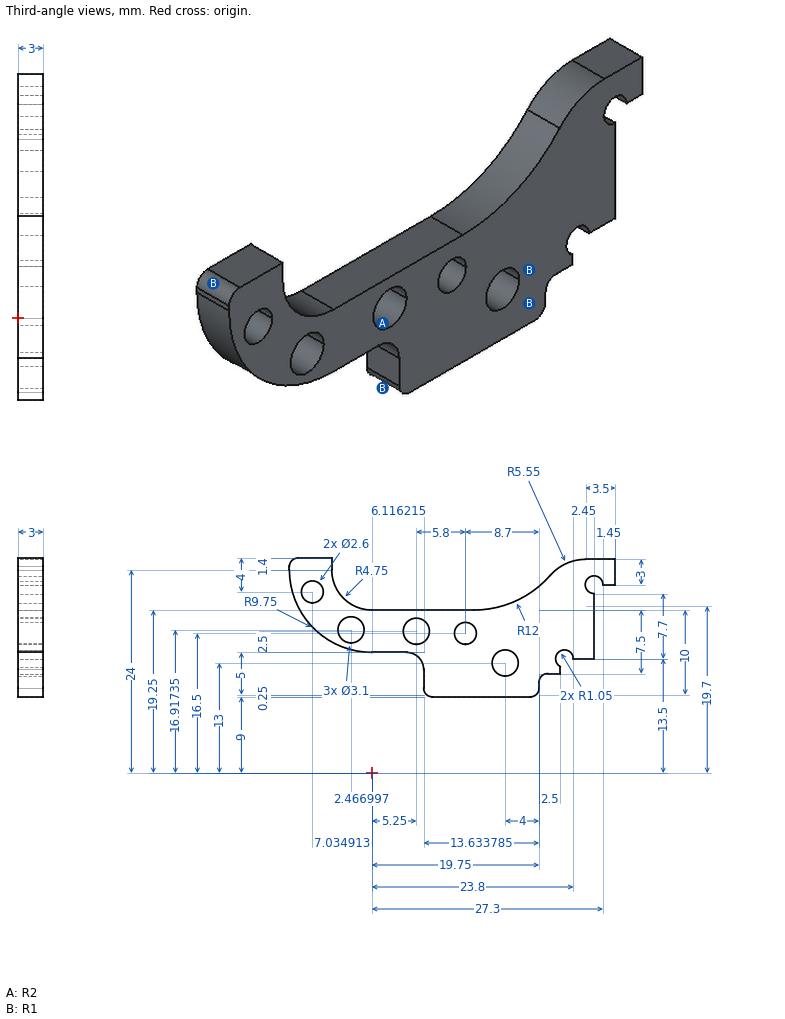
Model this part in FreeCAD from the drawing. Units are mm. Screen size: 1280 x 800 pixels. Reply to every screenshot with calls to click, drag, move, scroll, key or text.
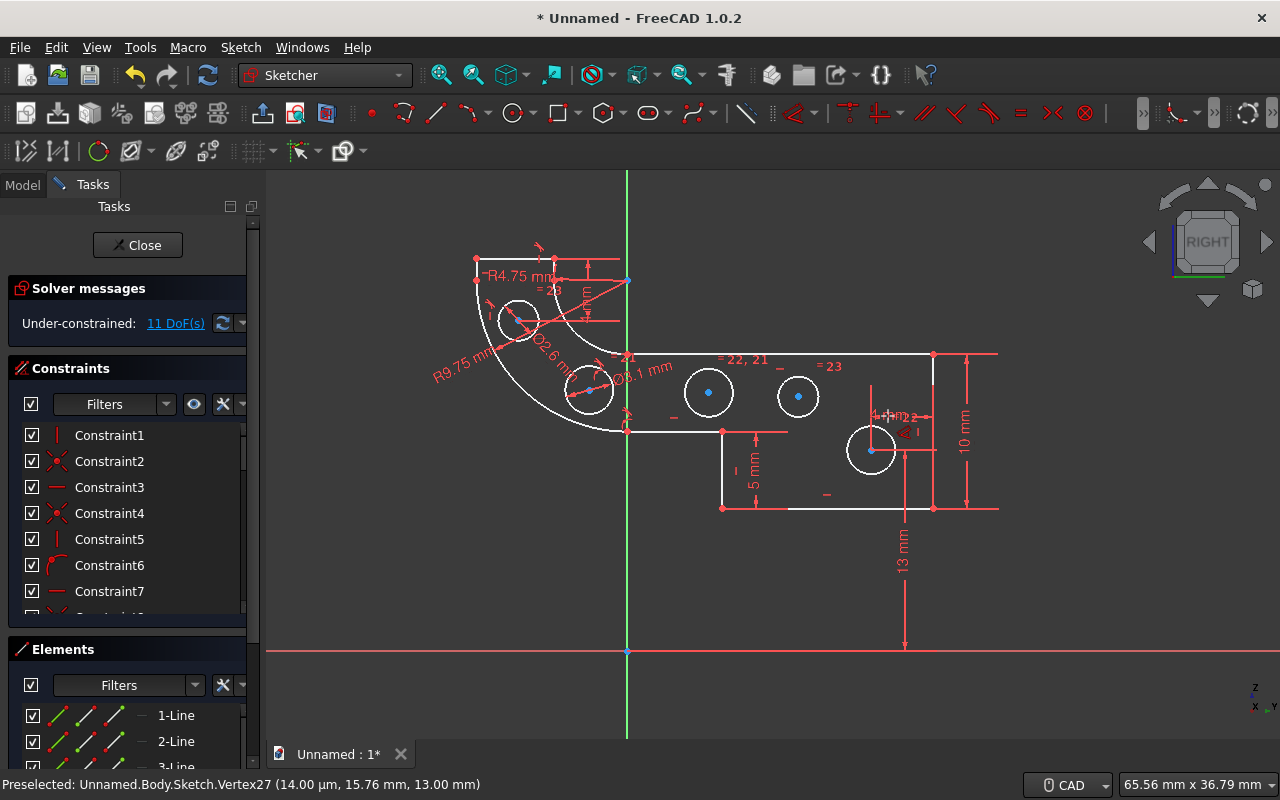
scroll(554, 270, up, 4)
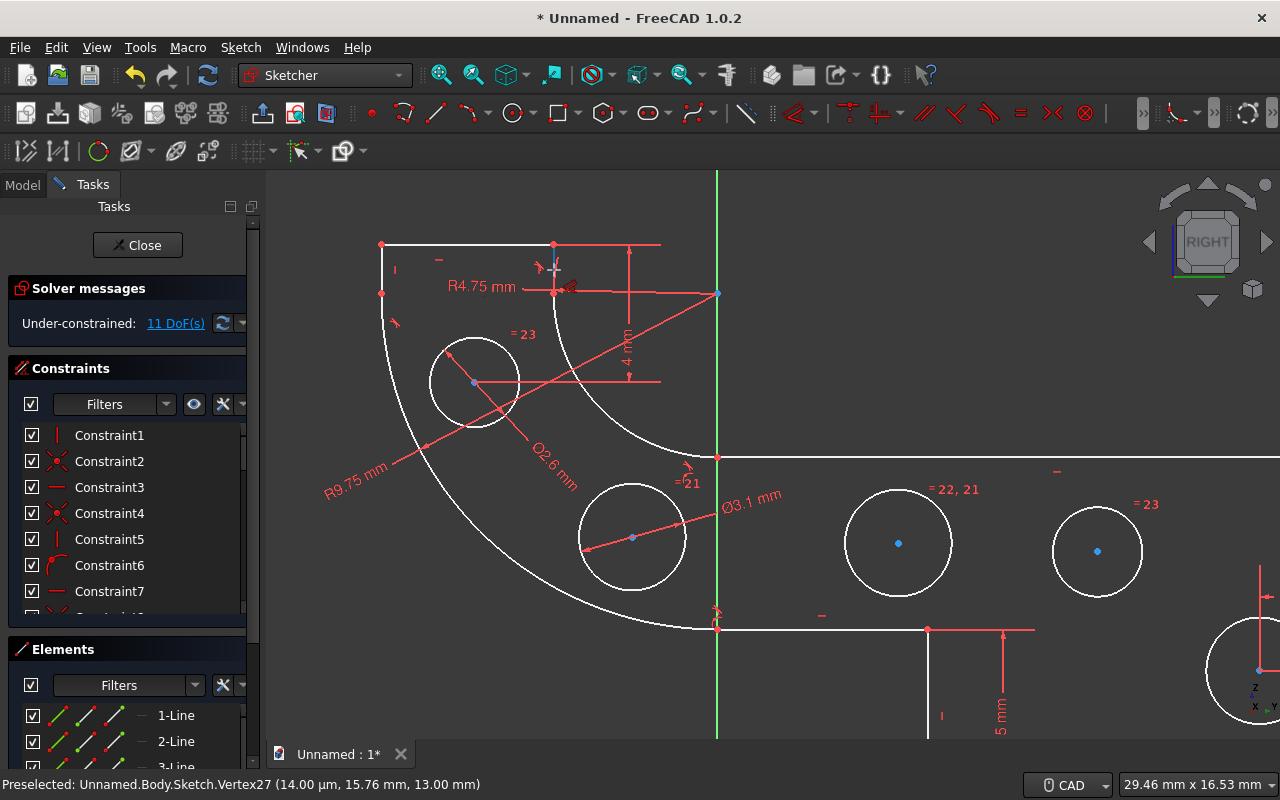
click(554, 269)
click(520, 258)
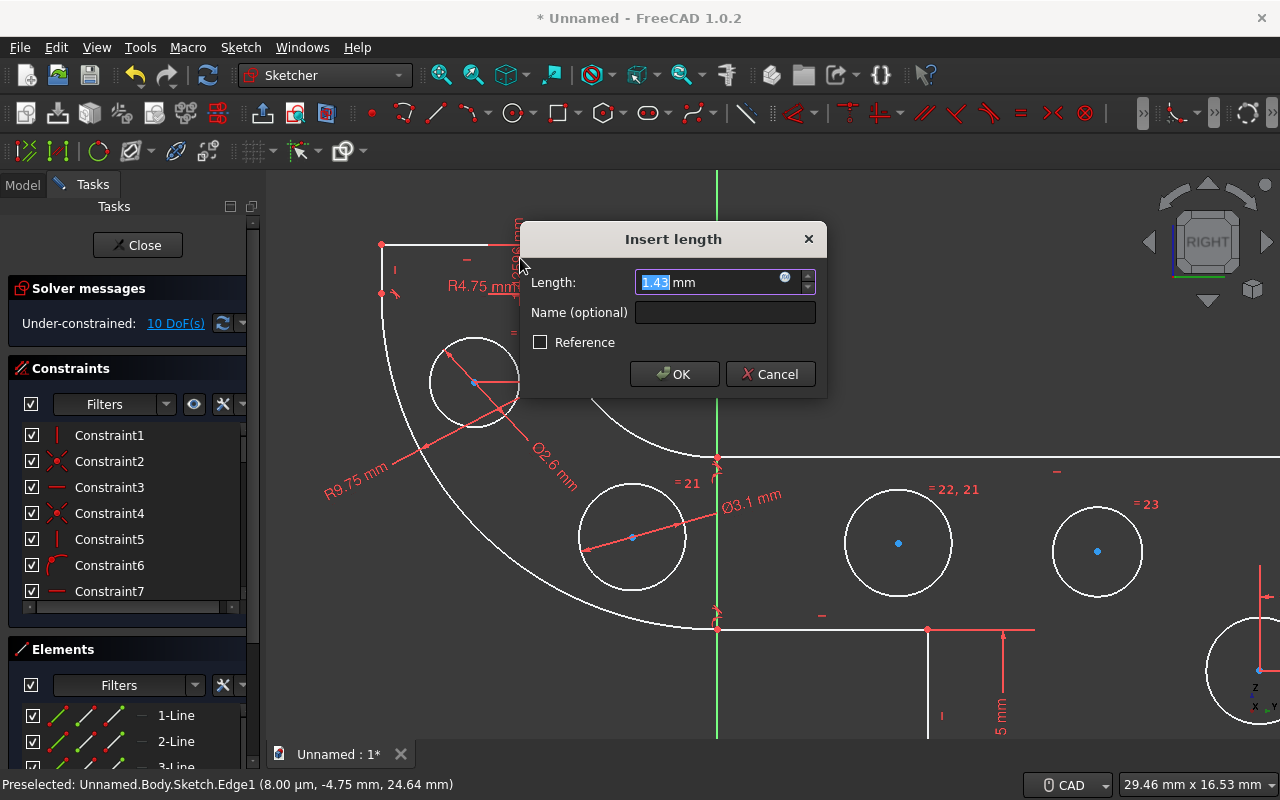
text(1.4)
key(Return)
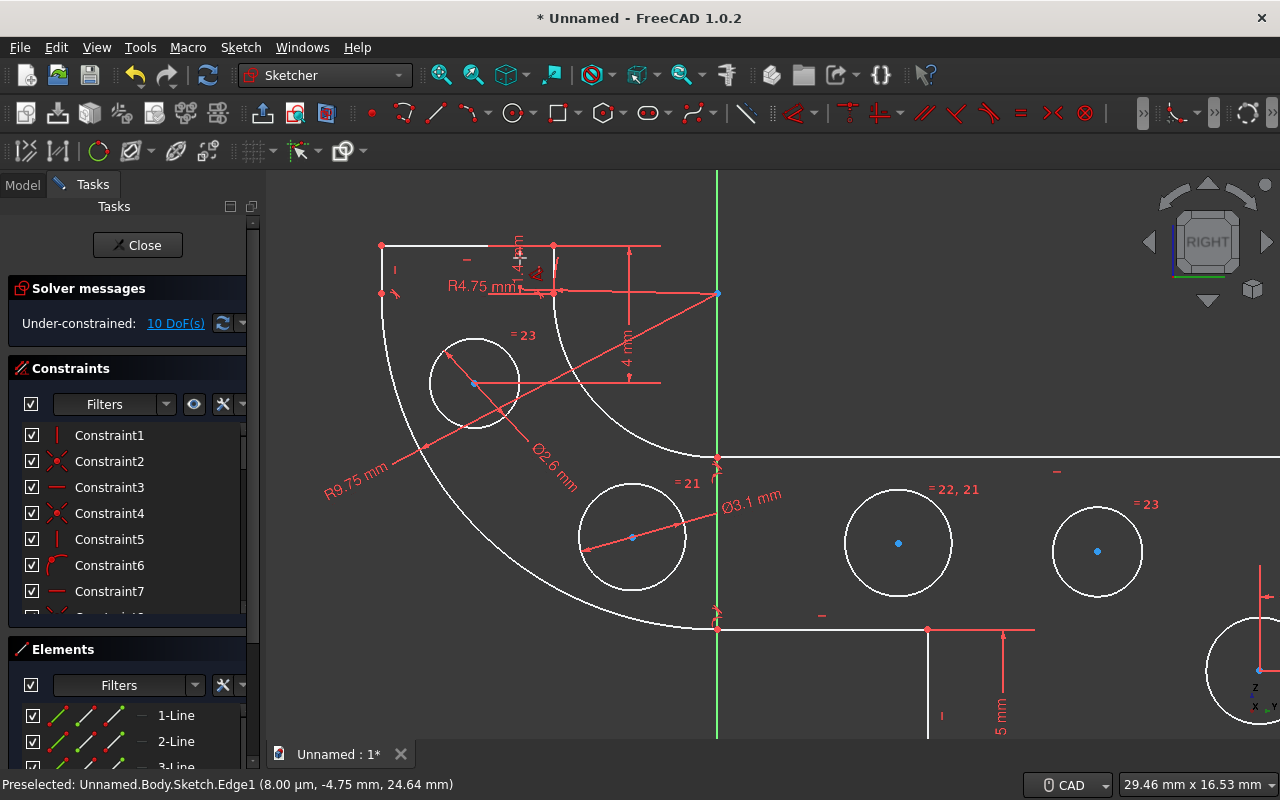
click(554, 294)
click(520, 502)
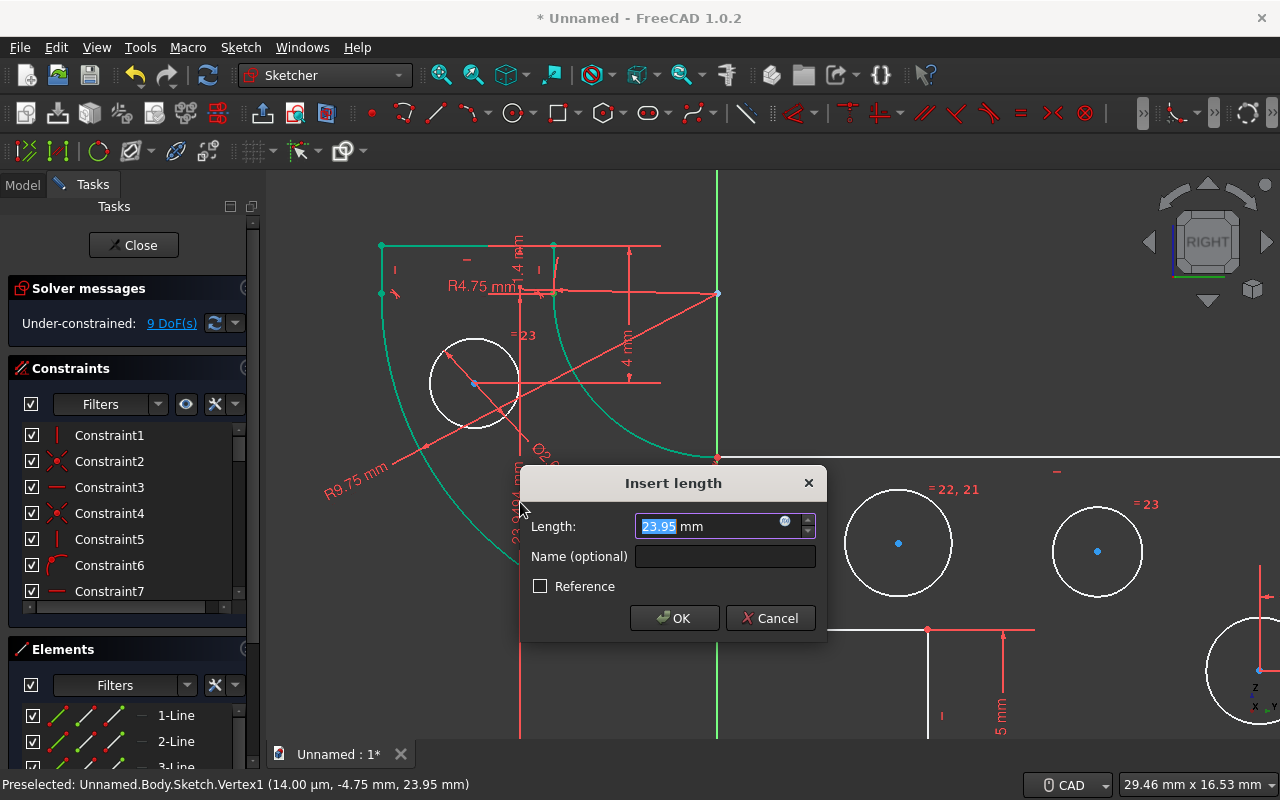
text(24)
key(Return)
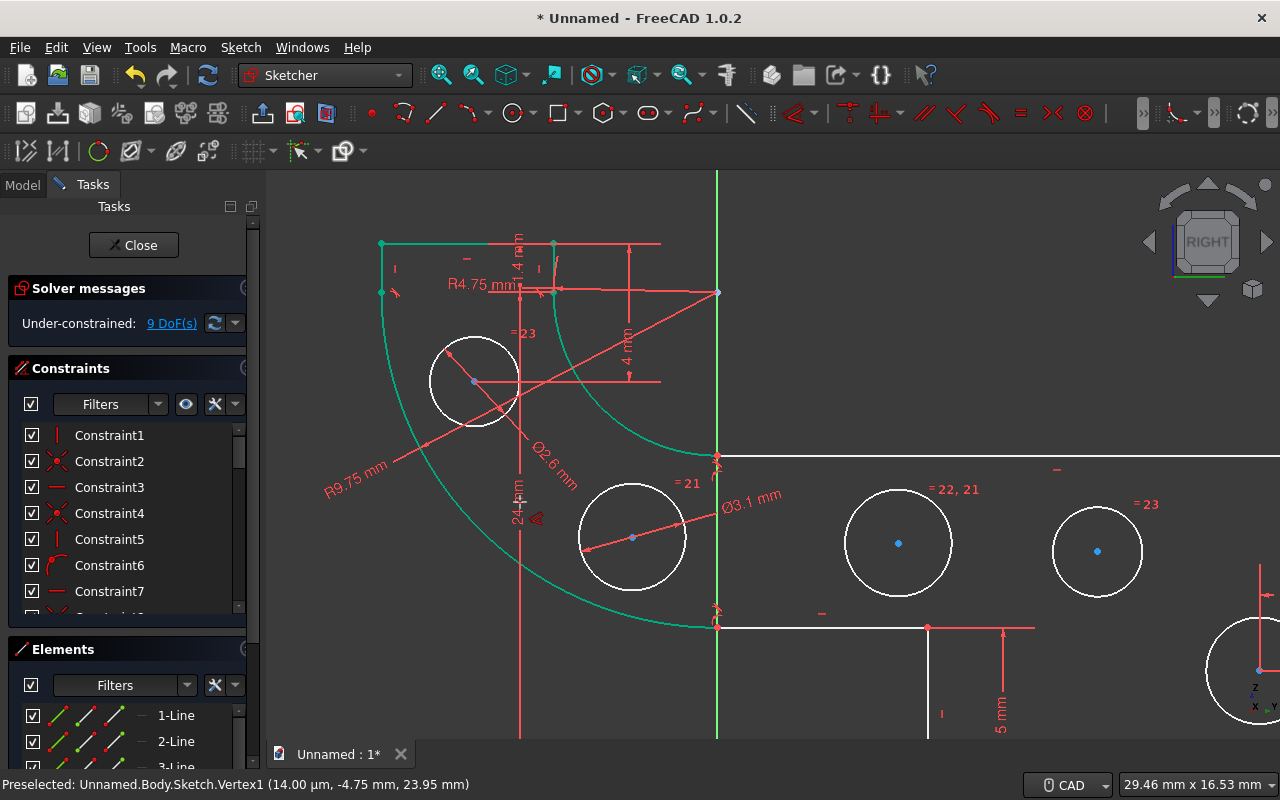
click(898, 543)
click(849, 485)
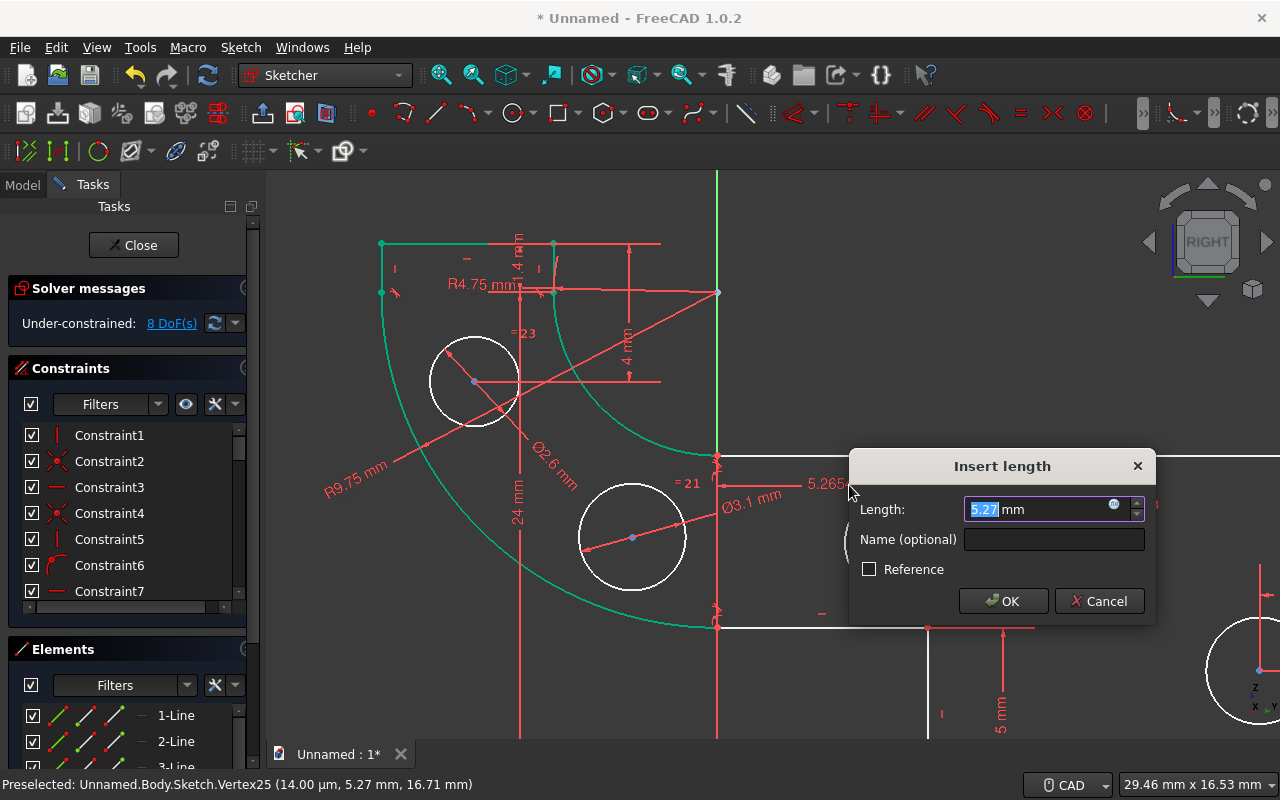
text(5.25)
key(Return)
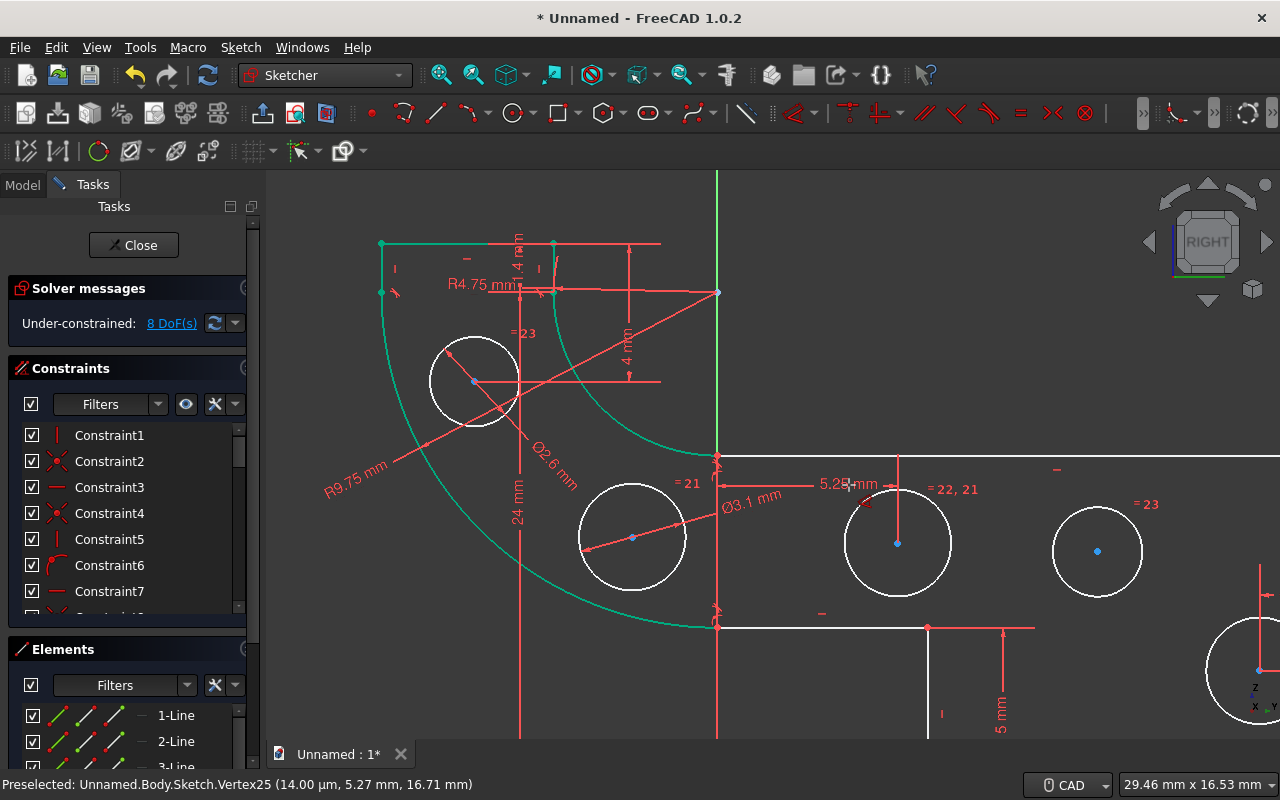
click(1098, 552)
click(683, 595)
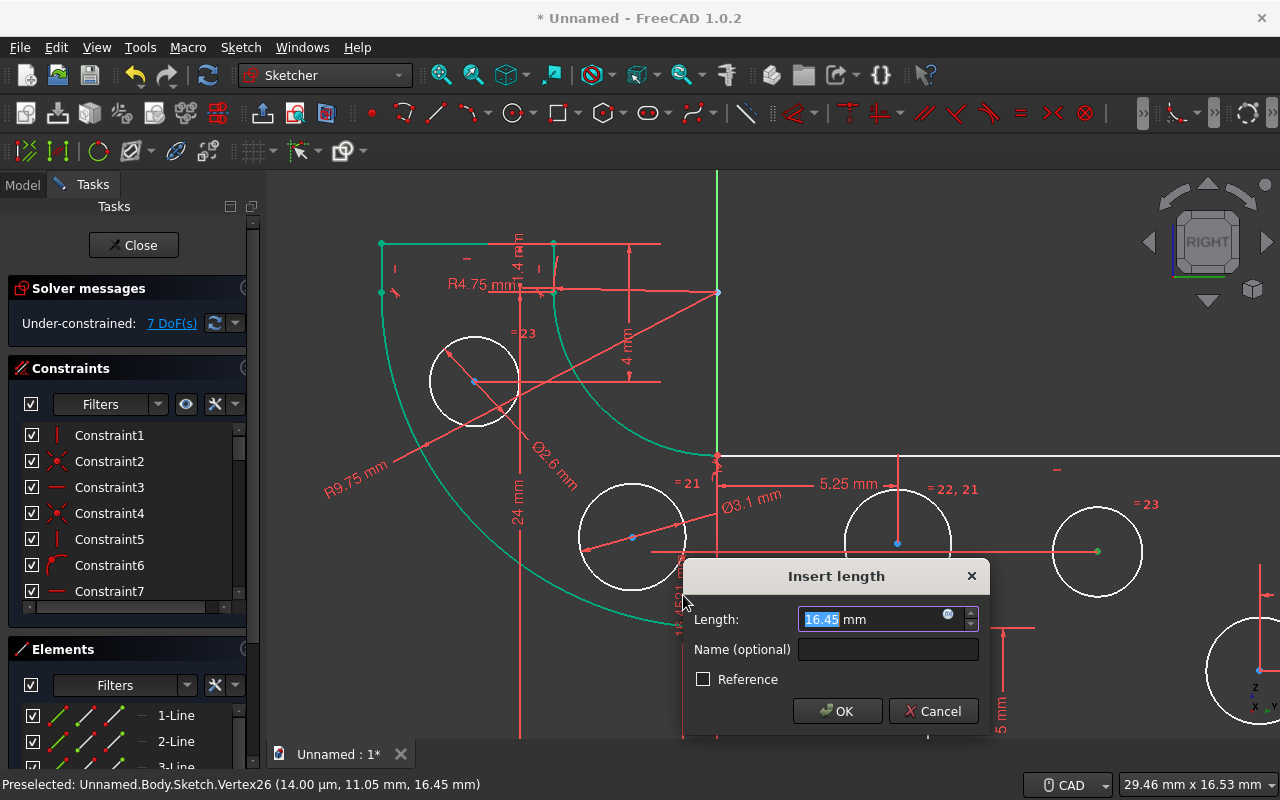
text(16.5)
key(Return)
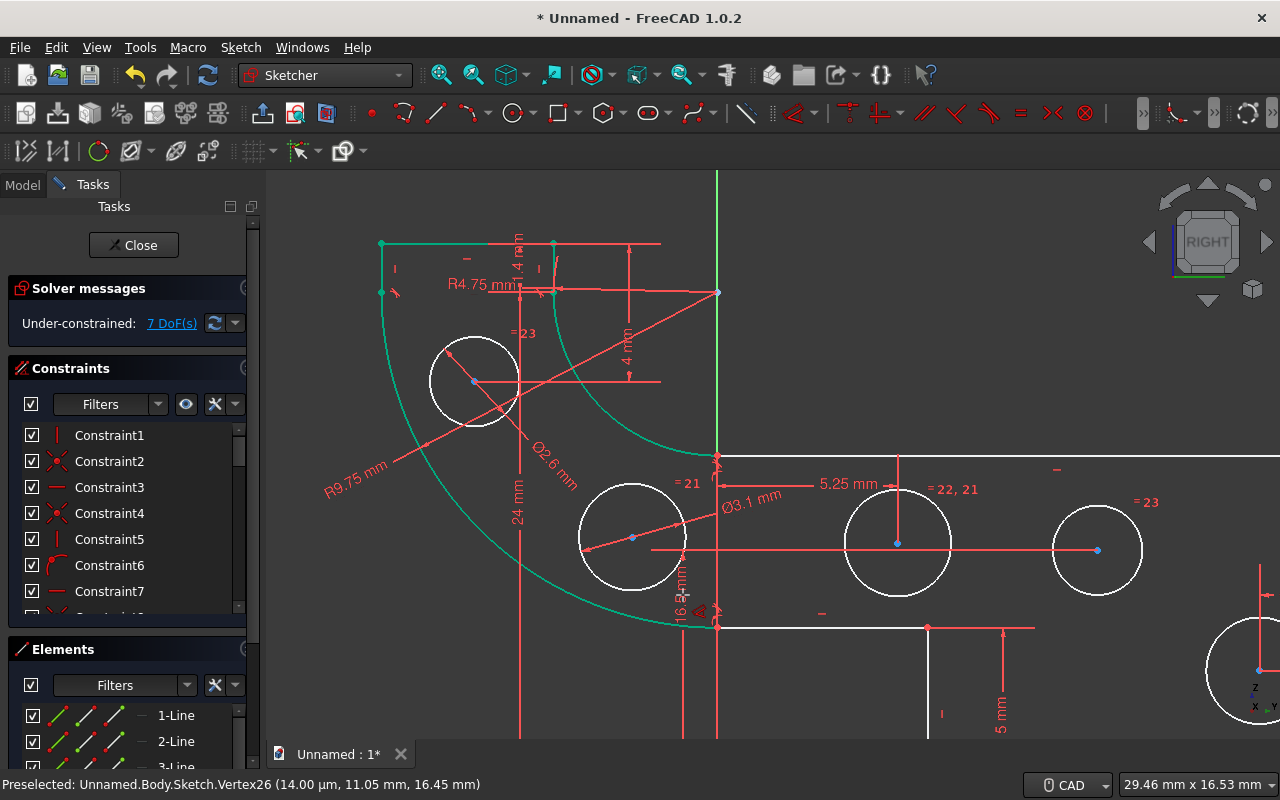
click(928, 628)